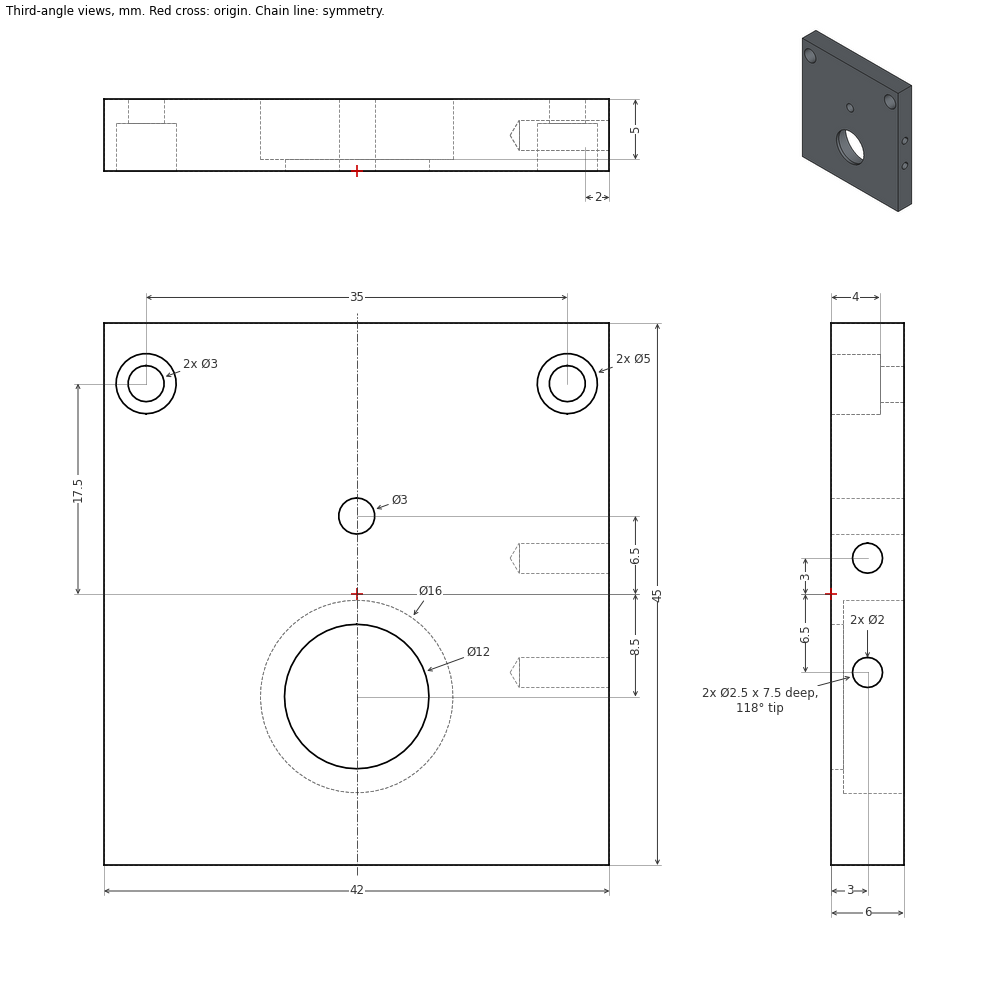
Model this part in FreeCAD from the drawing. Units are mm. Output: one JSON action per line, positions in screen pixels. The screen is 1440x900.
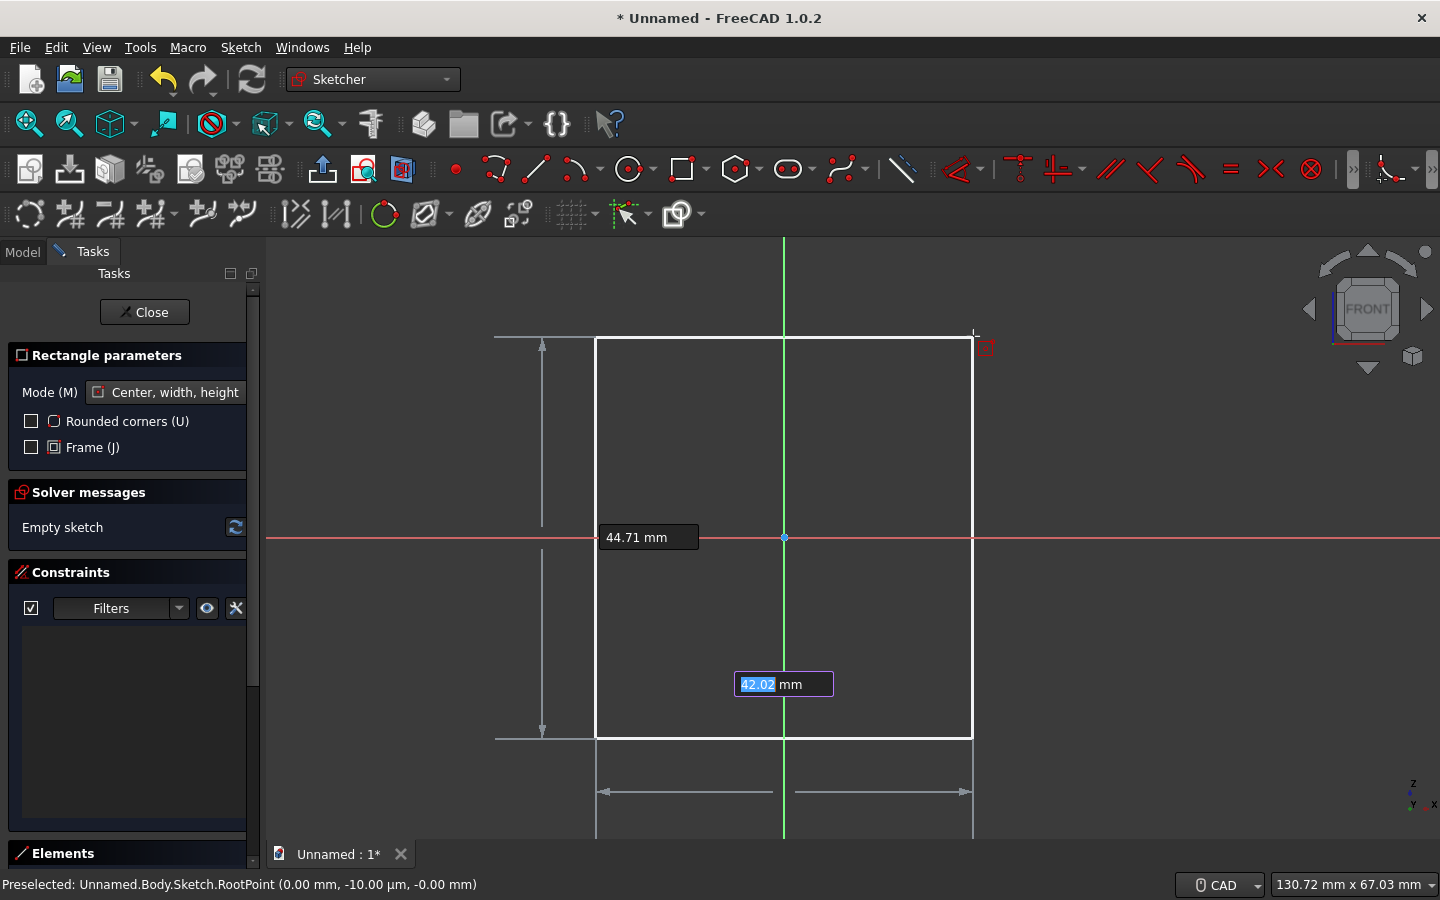
{"action": "type", "text": "42"}
{"action": "key", "text": "Tab"}
{"action": "type", "text": "45"}
{"action": "key", "text": "Return"}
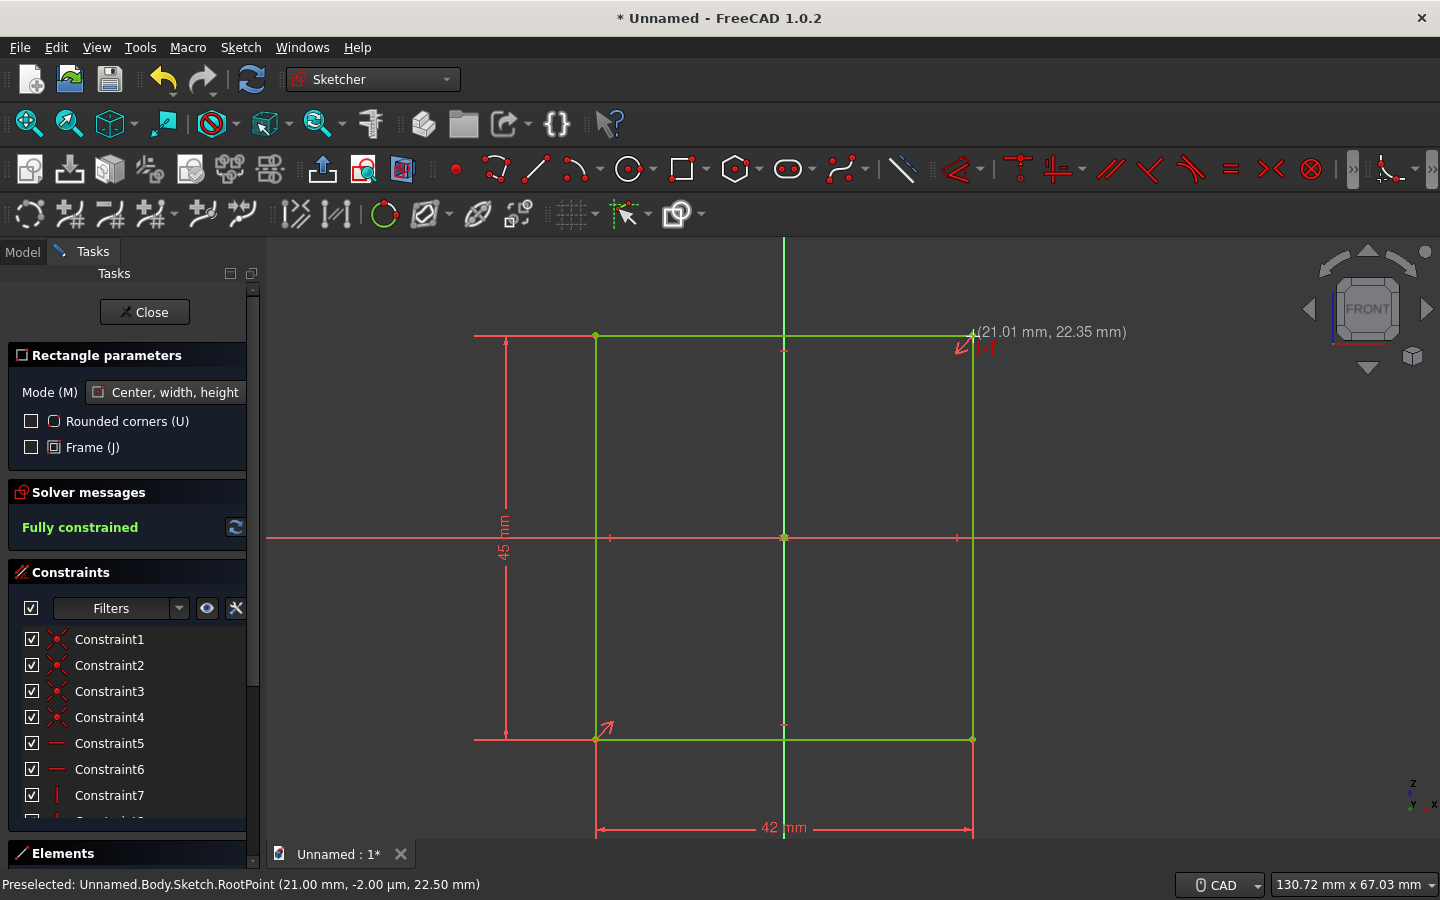
{"action": "key", "text": "g c"}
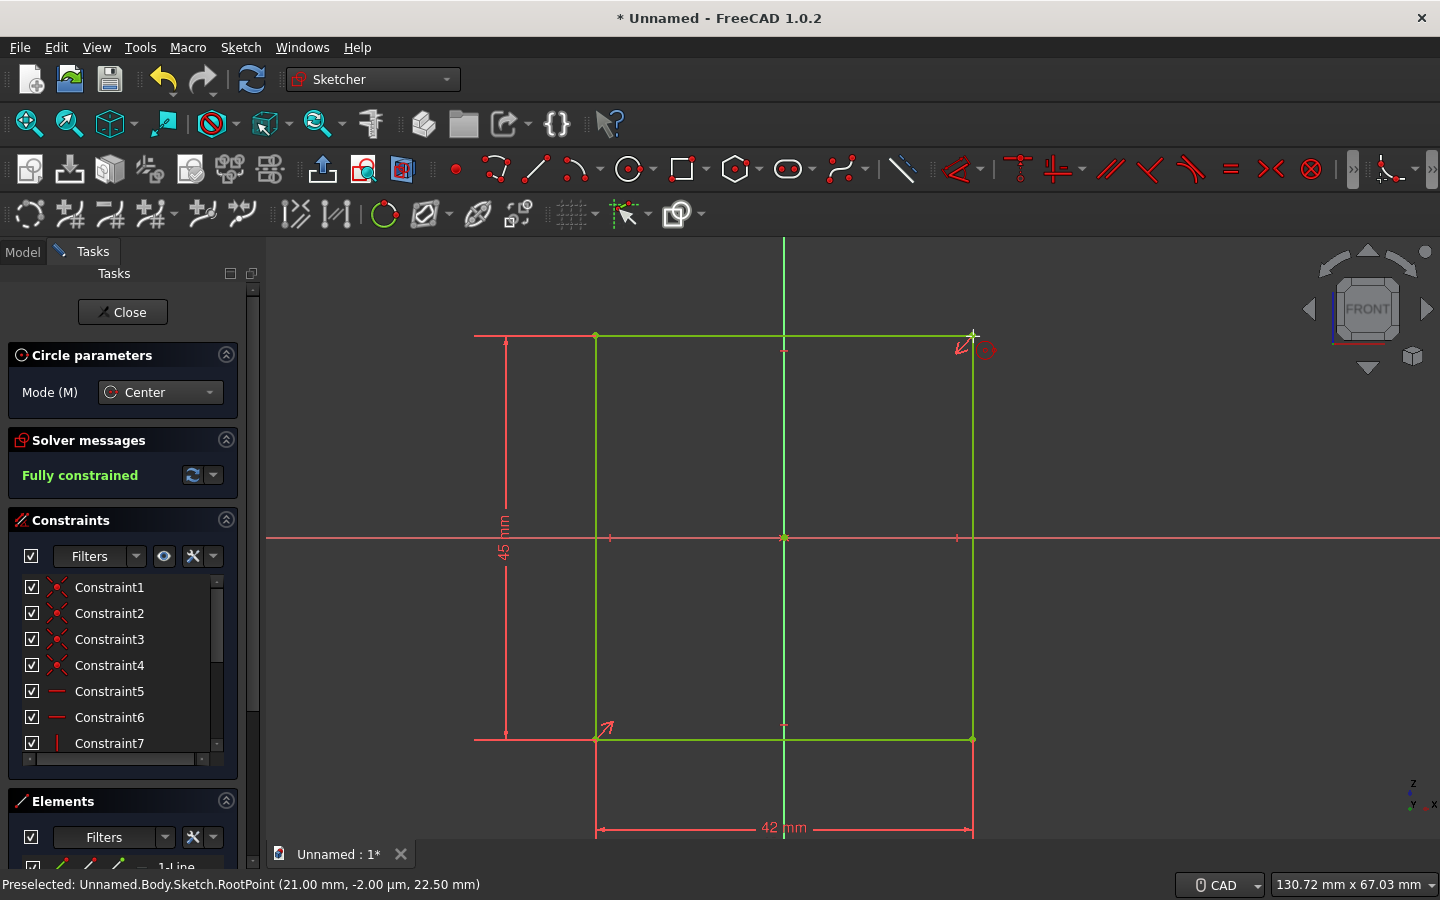
{"action": "scroll", "coordinate": [784, 479], "scroll_direction": "up", "scroll_amount": 3}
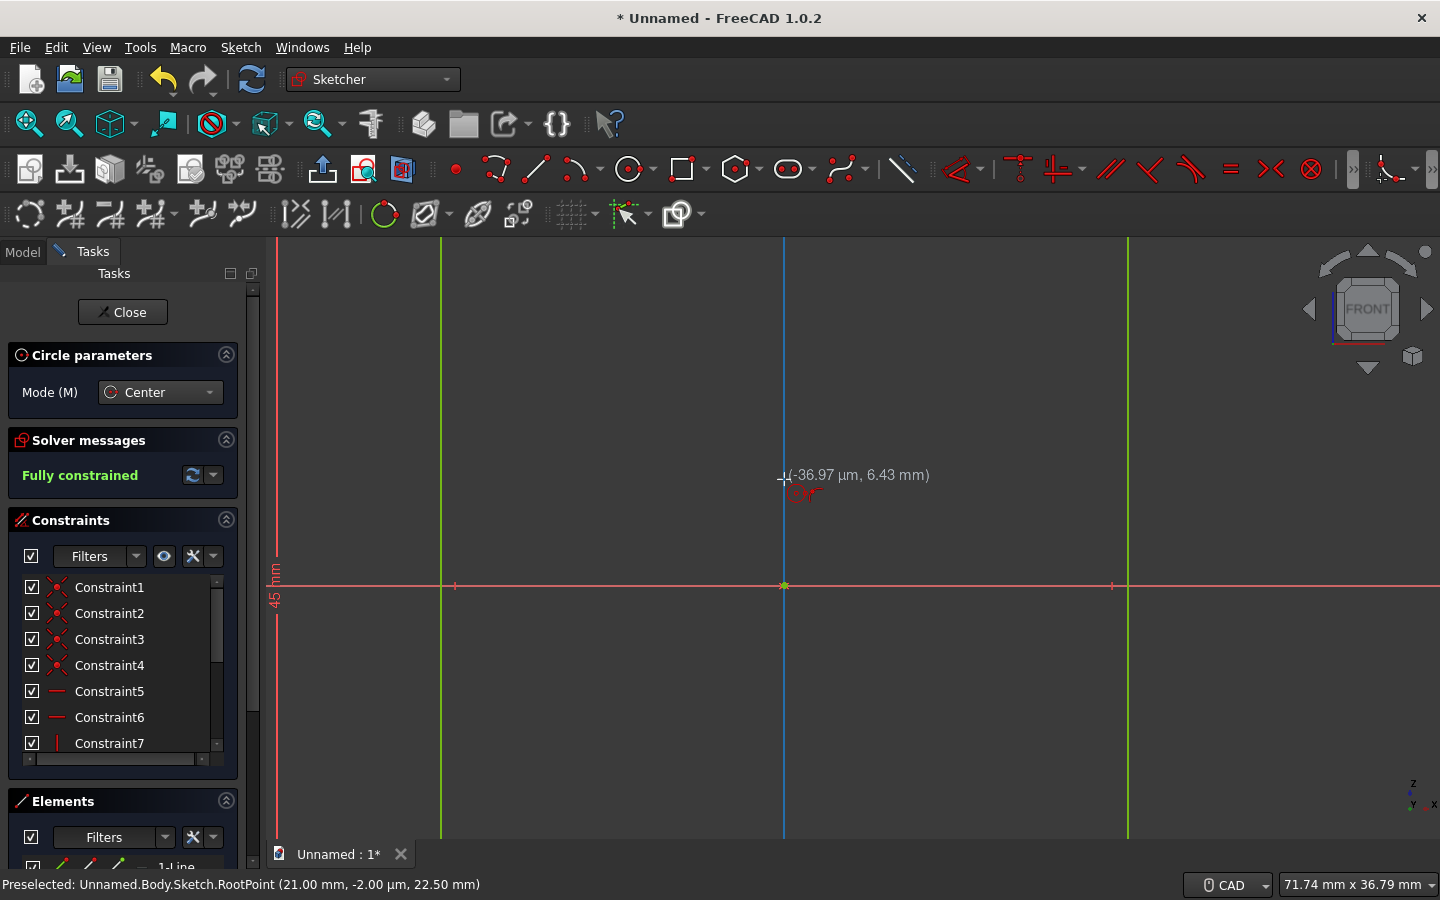
{"action": "left_click", "coordinate": [784, 479]}
{"action": "mouse_move", "coordinate": [802, 462]}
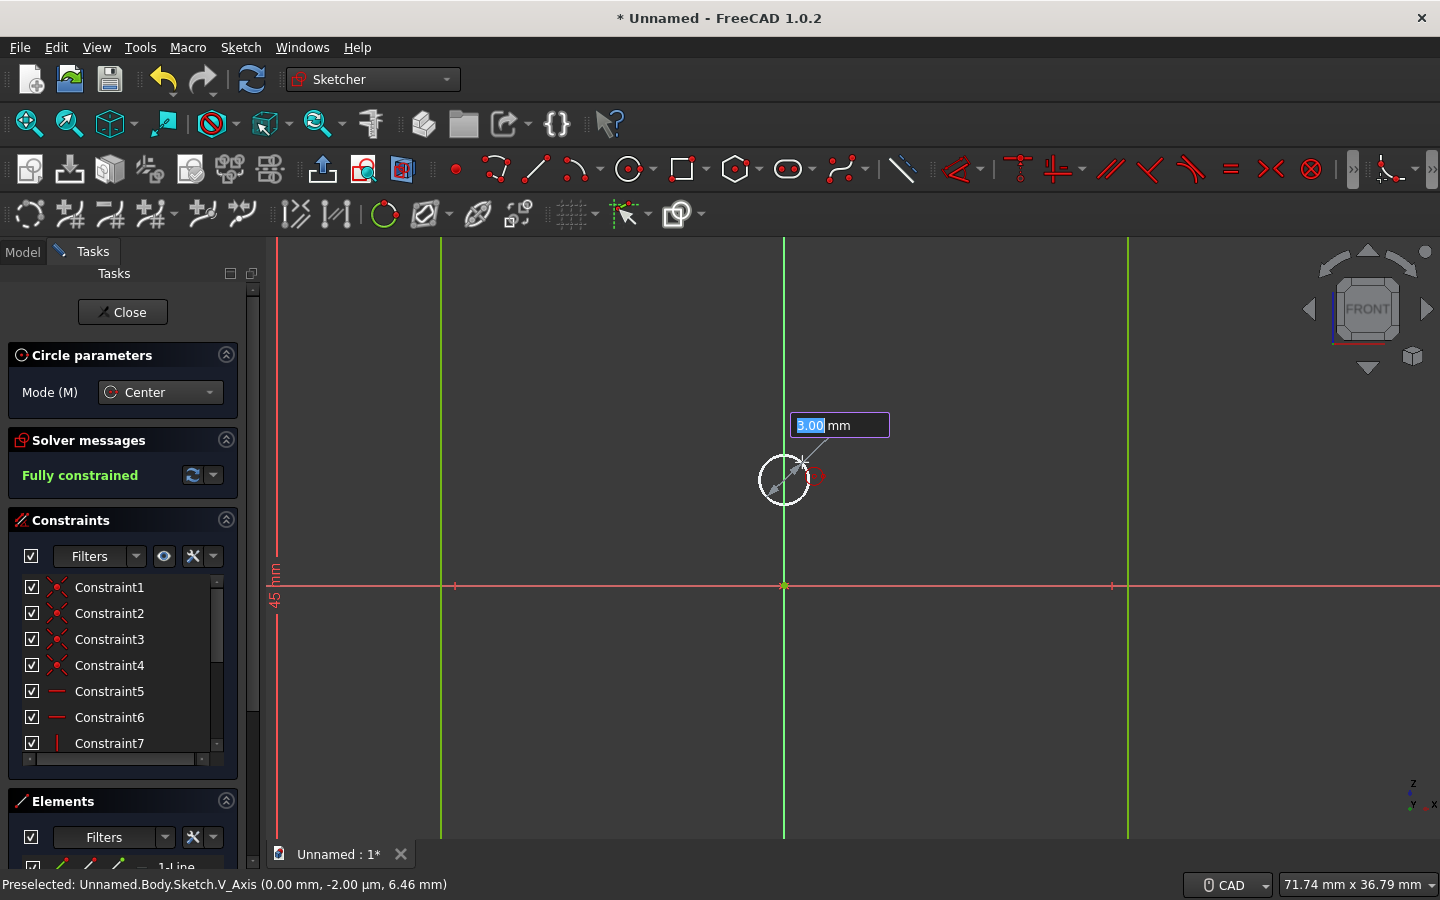
{"action": "type", "text": "3"}
{"action": "key", "text": "Return"}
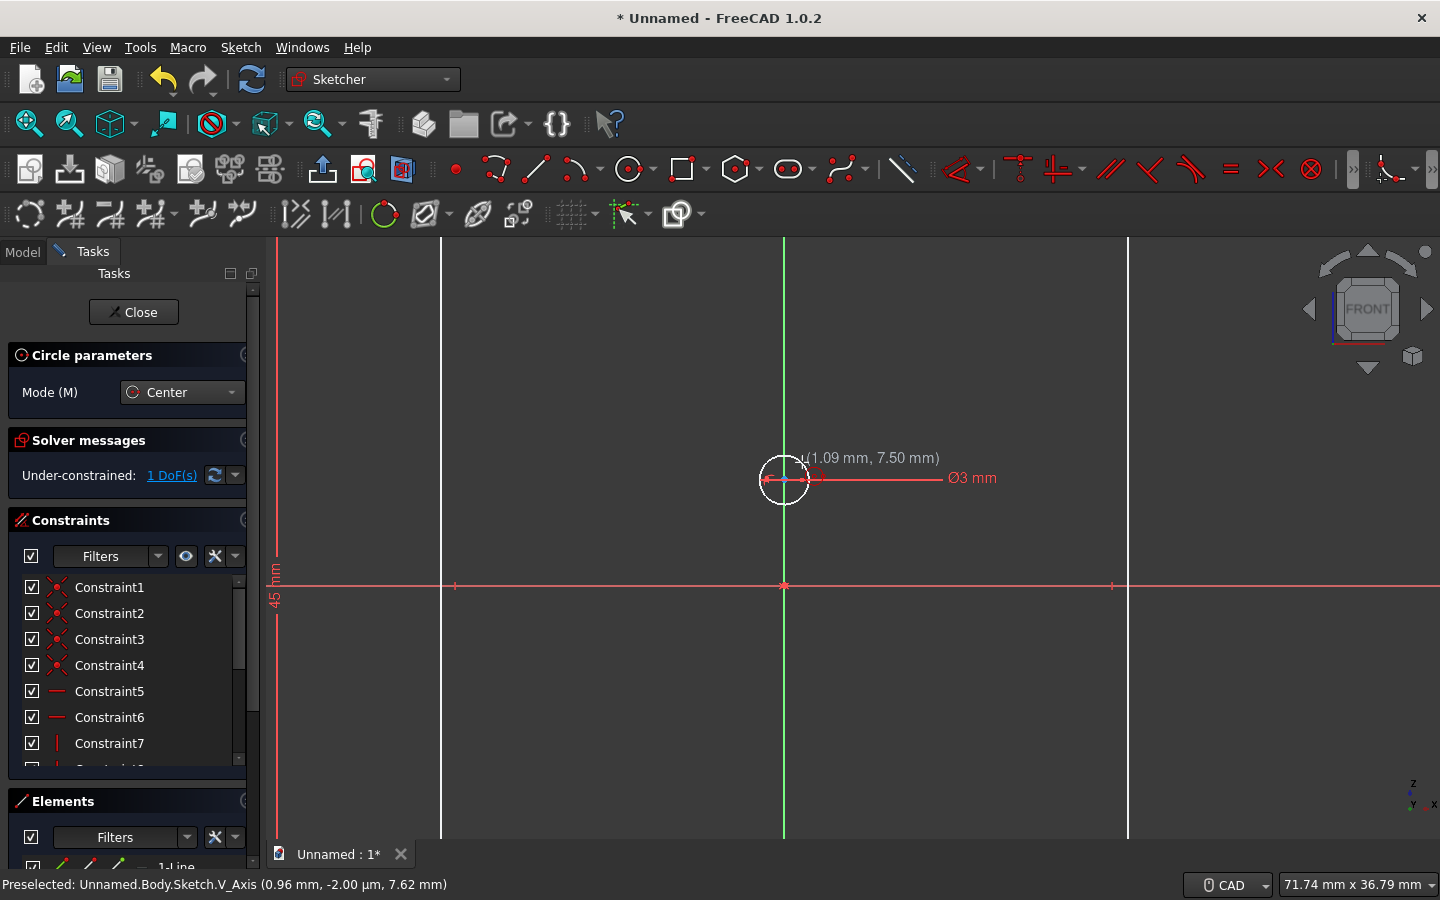
{"action": "left_click", "coordinate": [784, 725]}
{"action": "mouse_move", "coordinate": [854, 655]}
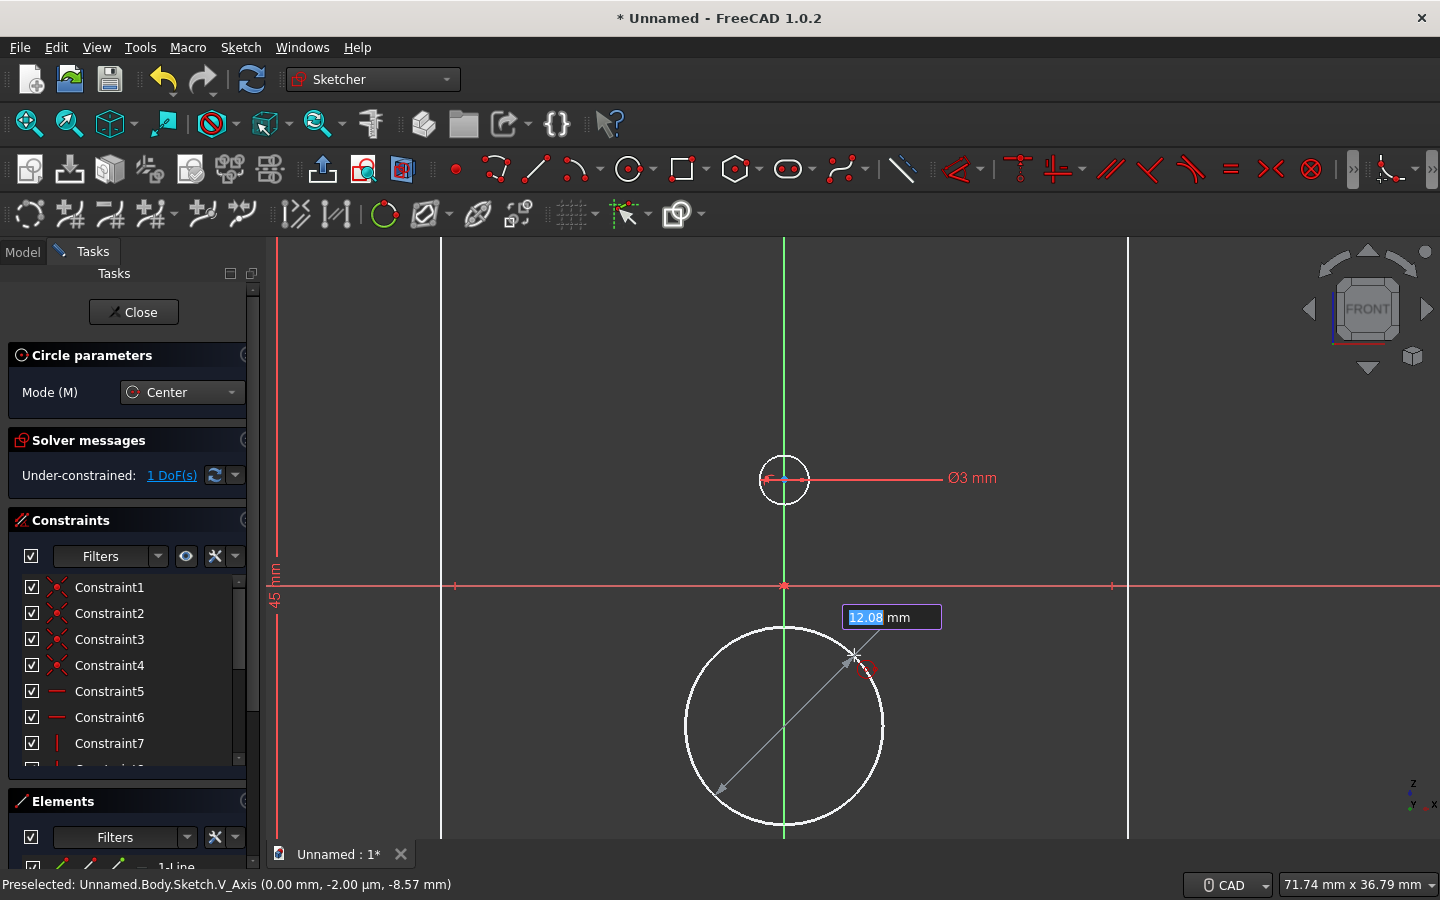
{"action": "type", "text": "12"}
{"action": "key", "text": "Return"}
{"action": "key", "text": "Escape"}